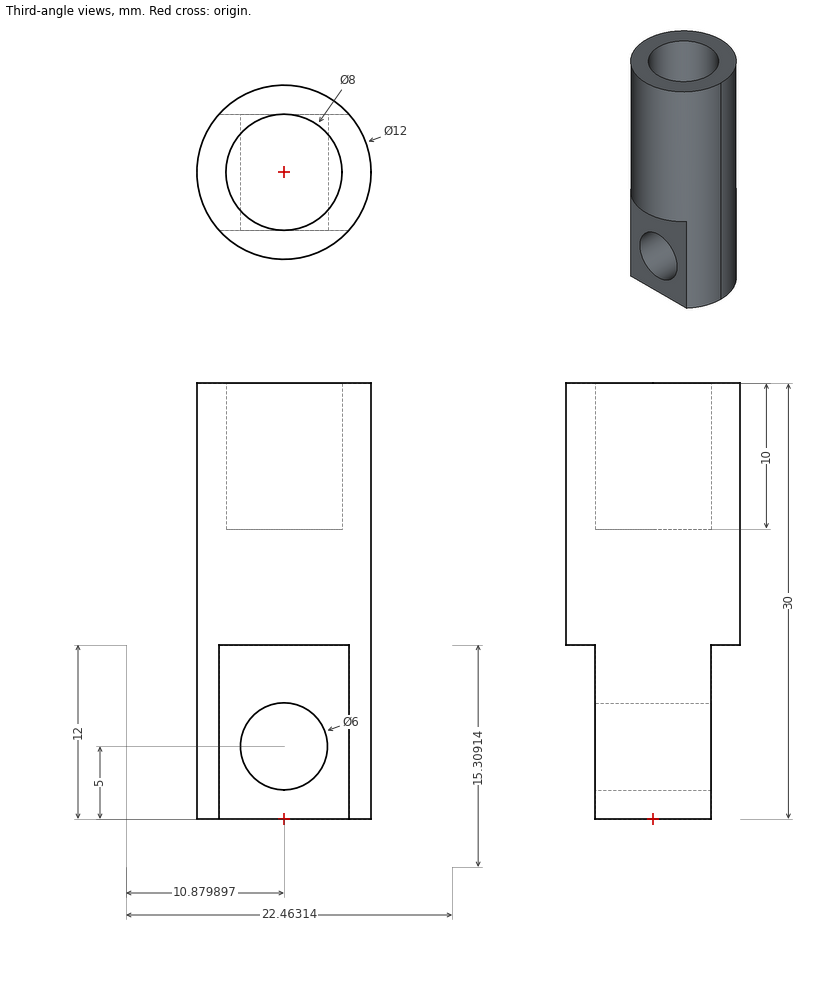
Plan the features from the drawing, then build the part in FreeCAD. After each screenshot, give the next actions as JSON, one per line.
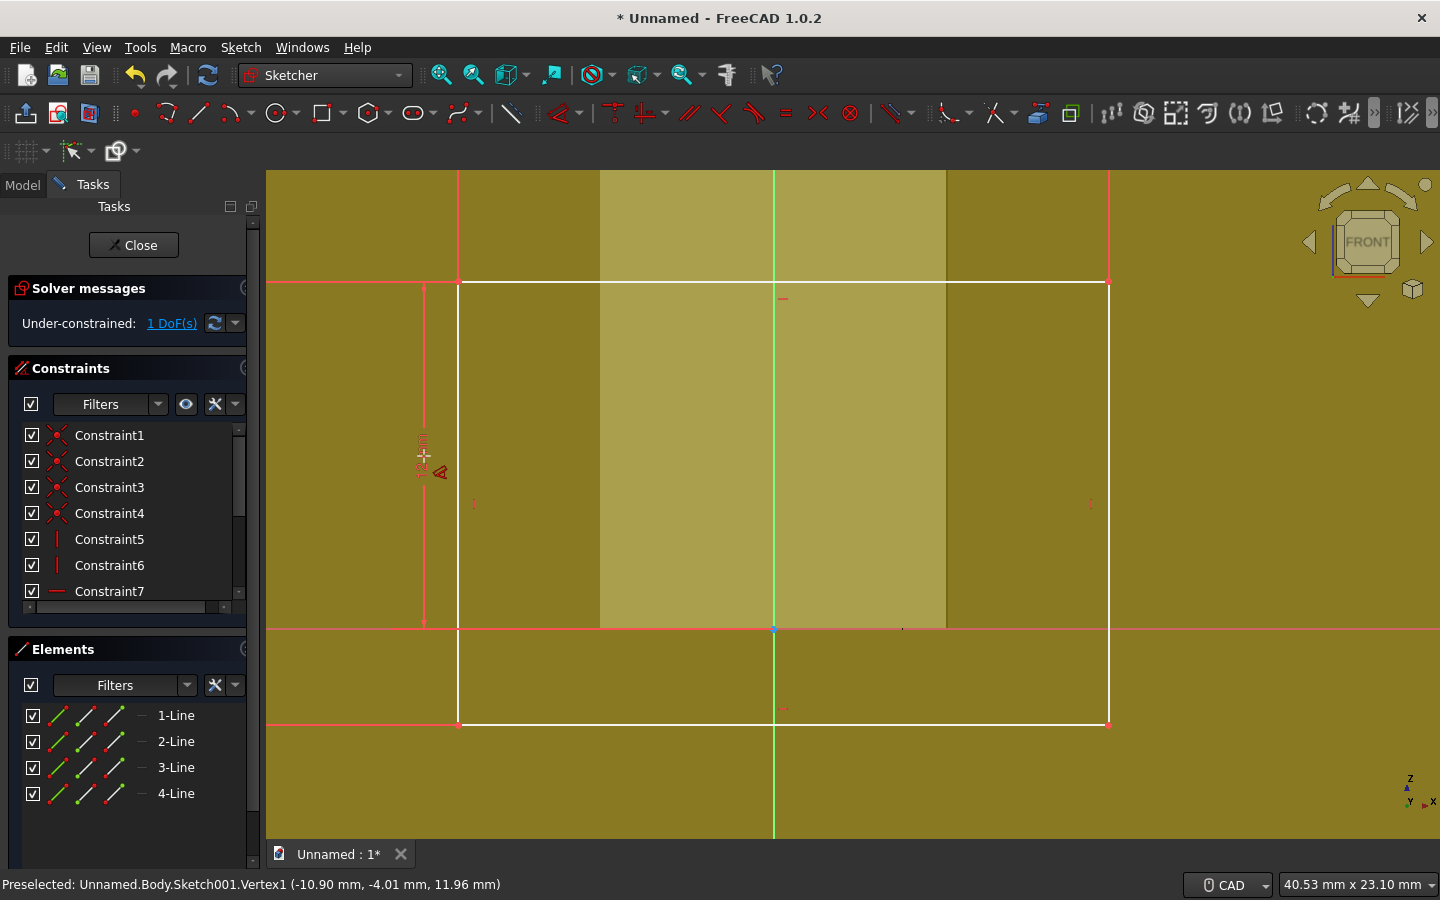
{"action": "left_click", "coordinate": [458, 282]}
{"action": "left_click", "coordinate": [616, 248]}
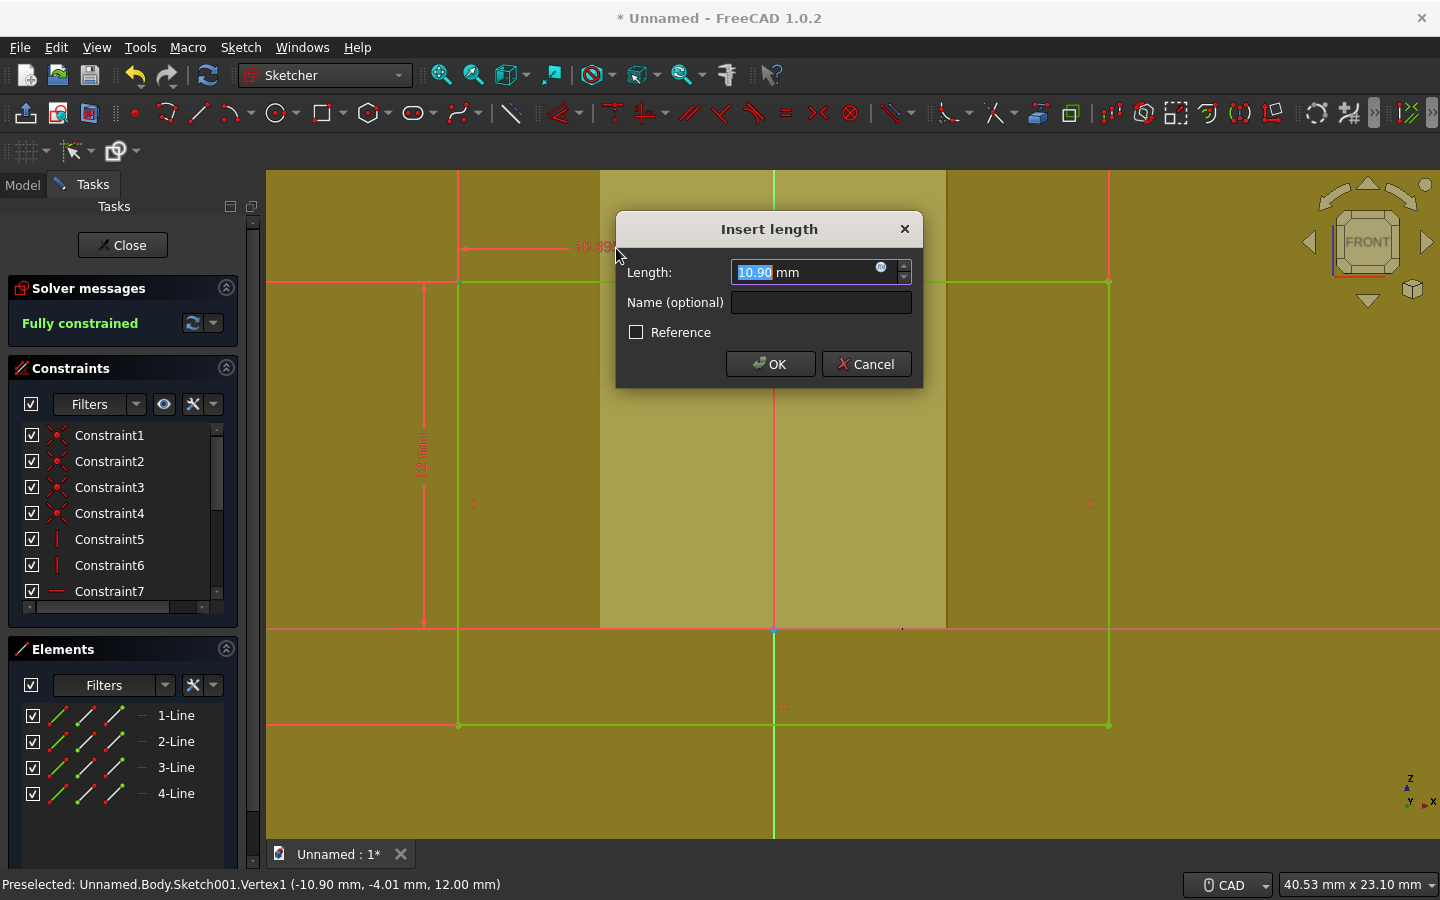
{"action": "type", "text": "10.879897"}
{"action": "key", "text": "Return"}
{"action": "key", "text": "Escape"}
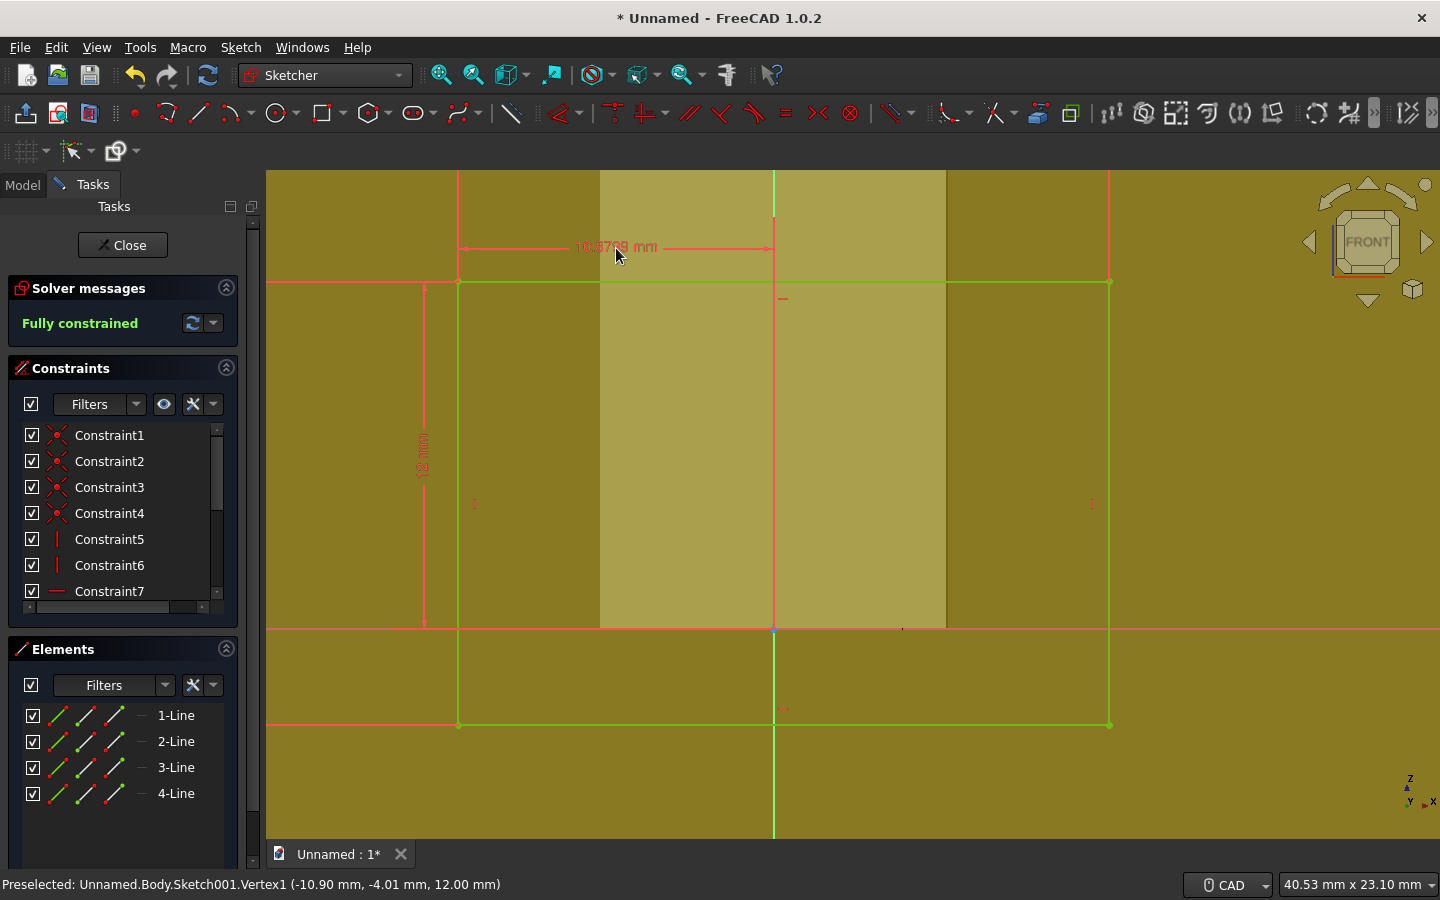
{"action": "left_click", "coordinate": [123, 245]}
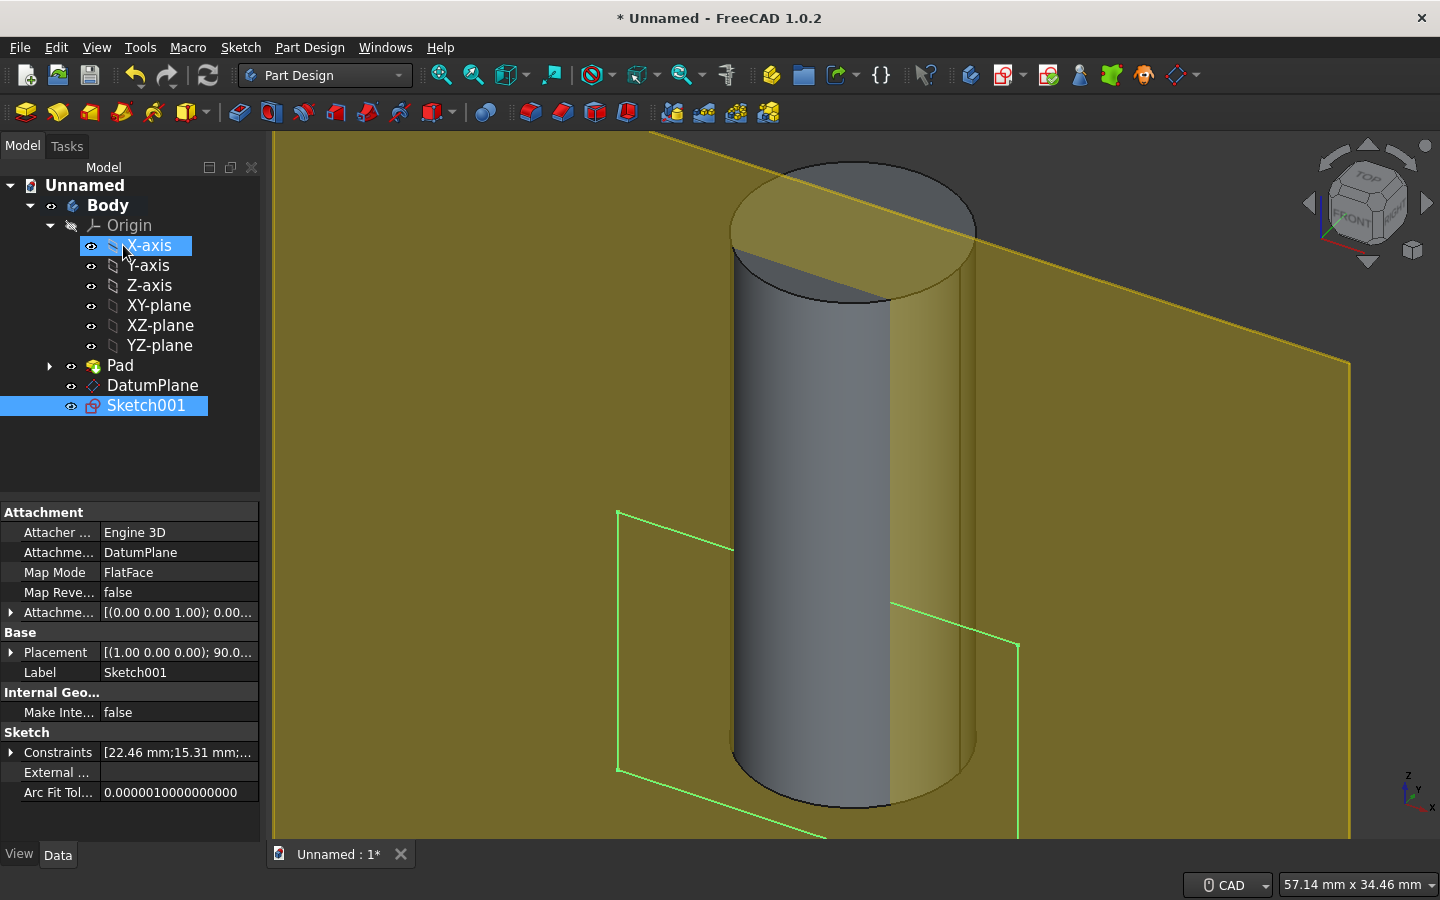
{"action": "left_click", "coordinate": [240, 112]}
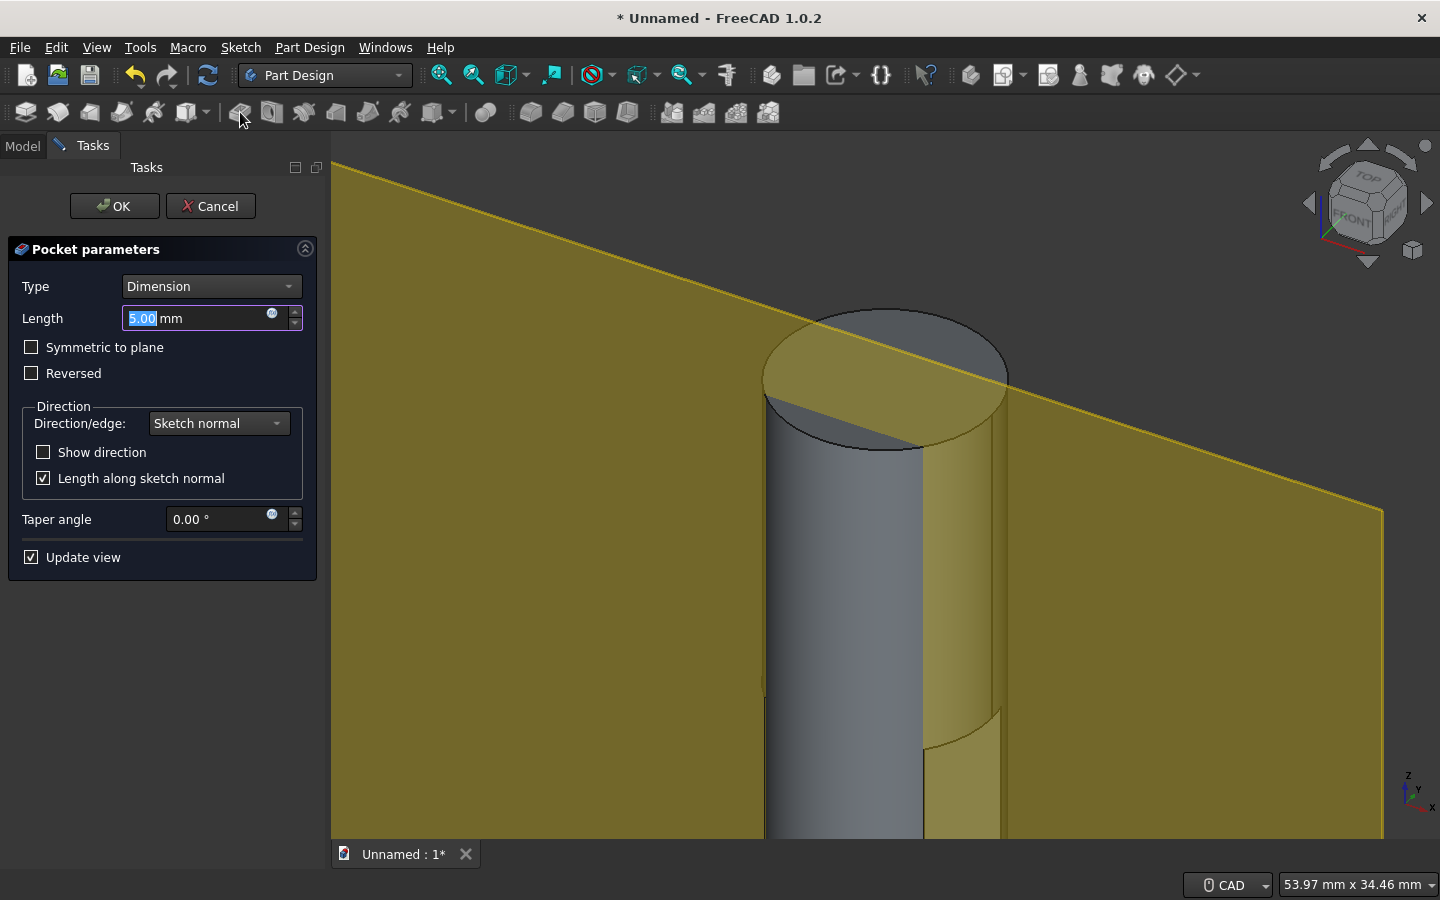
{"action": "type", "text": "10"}
{"action": "key", "text": "Tab"}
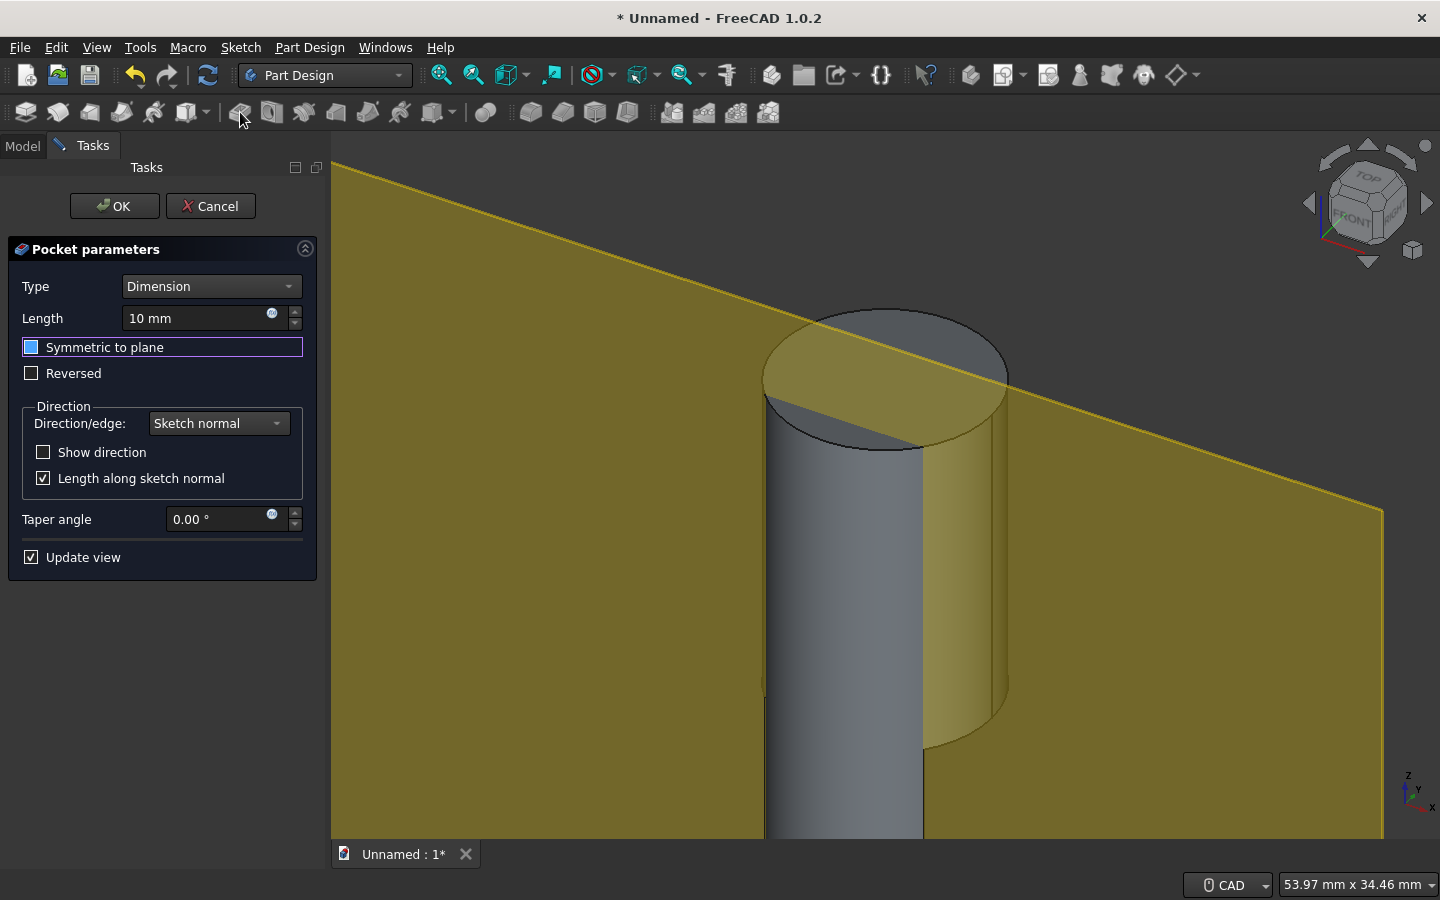
{"action": "left_click", "coordinate": [30, 373]}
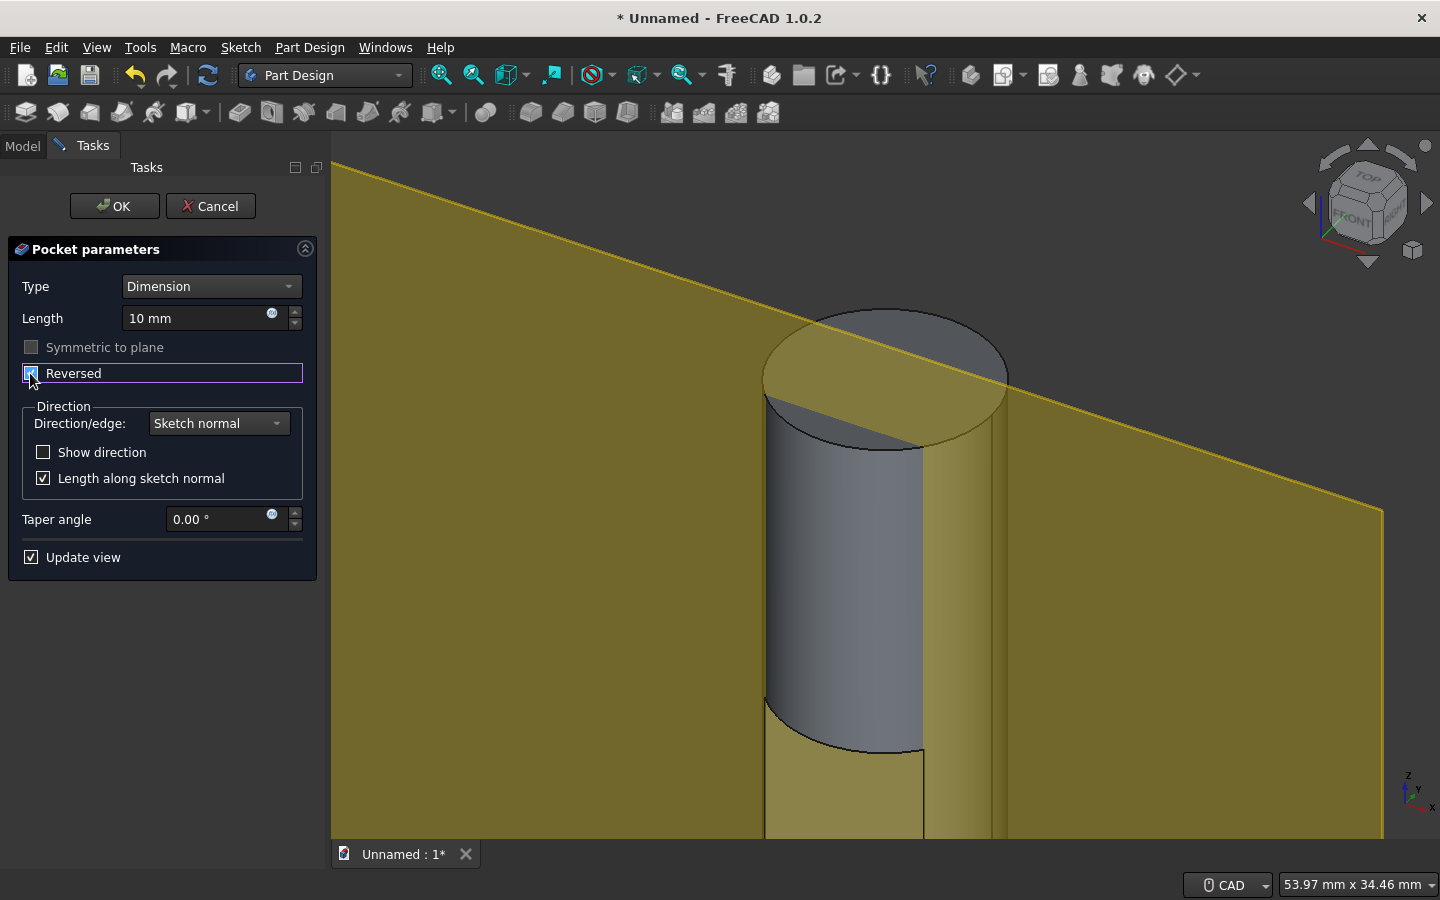
{"action": "left_click", "coordinate": [115, 206]}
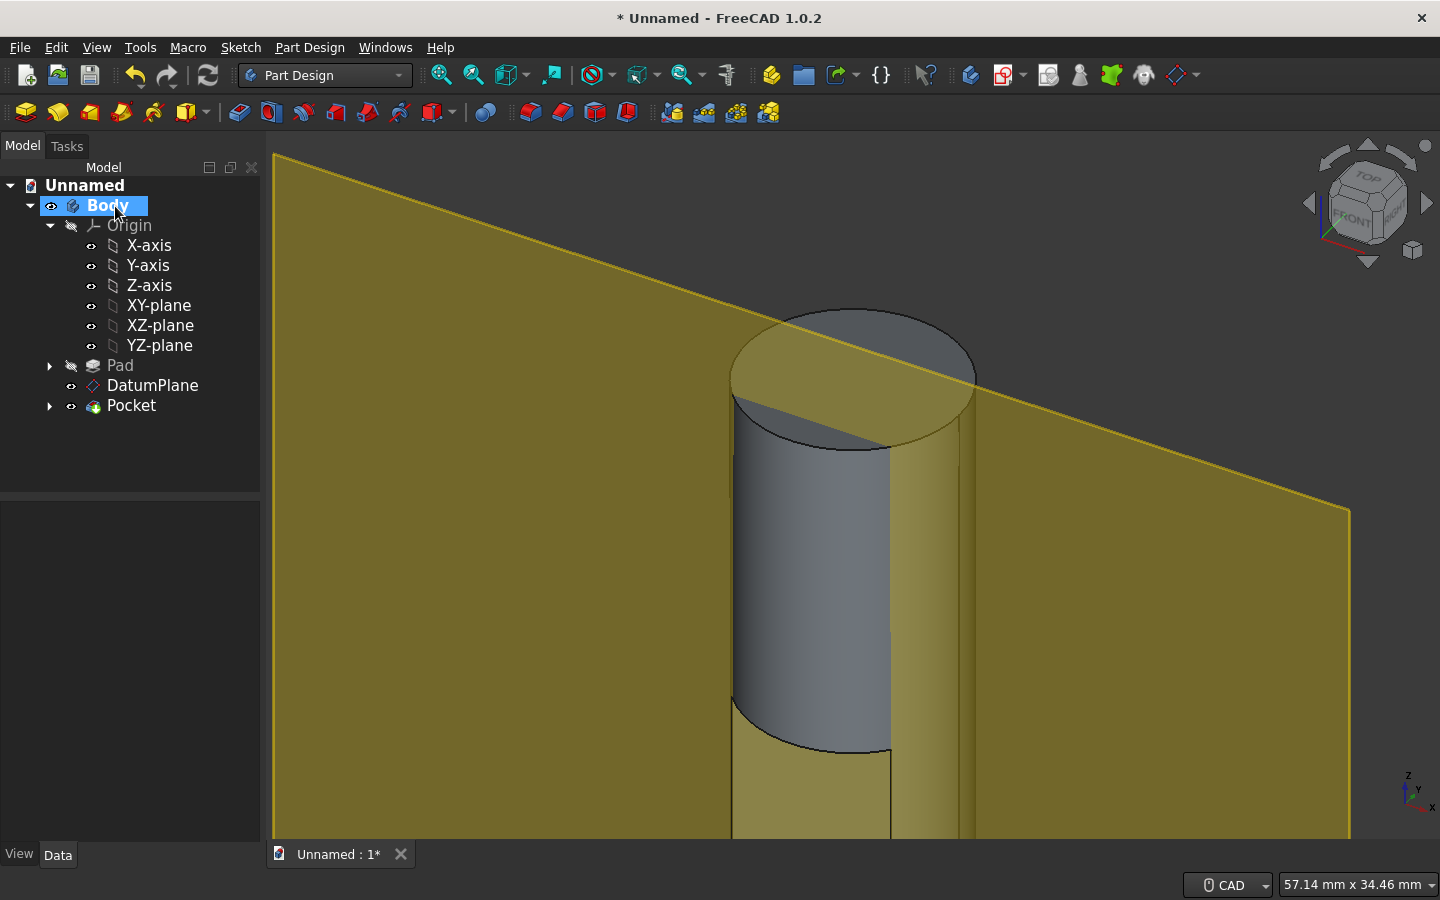
{"action": "left_click", "coordinate": [116, 386]}
{"action": "key", "text": "space"}